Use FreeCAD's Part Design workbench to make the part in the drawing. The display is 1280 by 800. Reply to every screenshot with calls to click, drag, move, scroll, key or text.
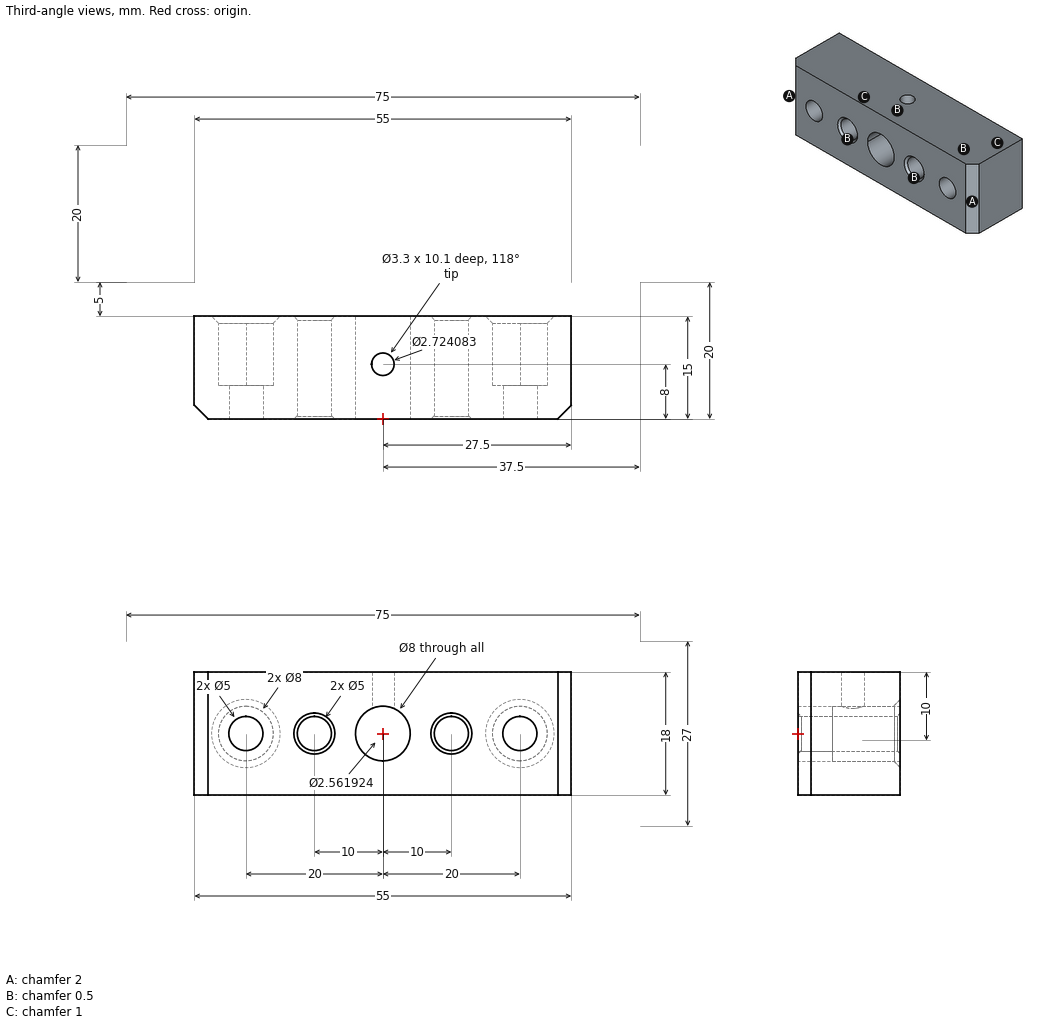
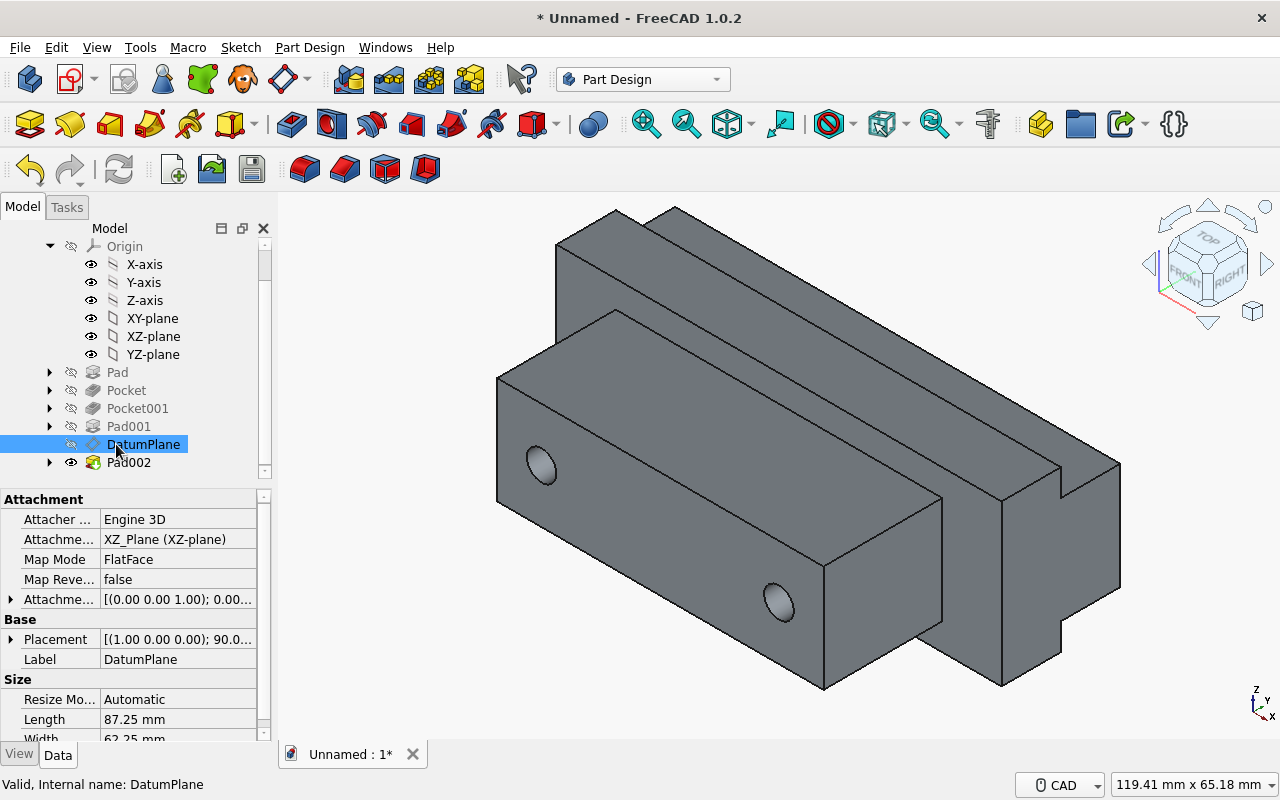
click(648, 124)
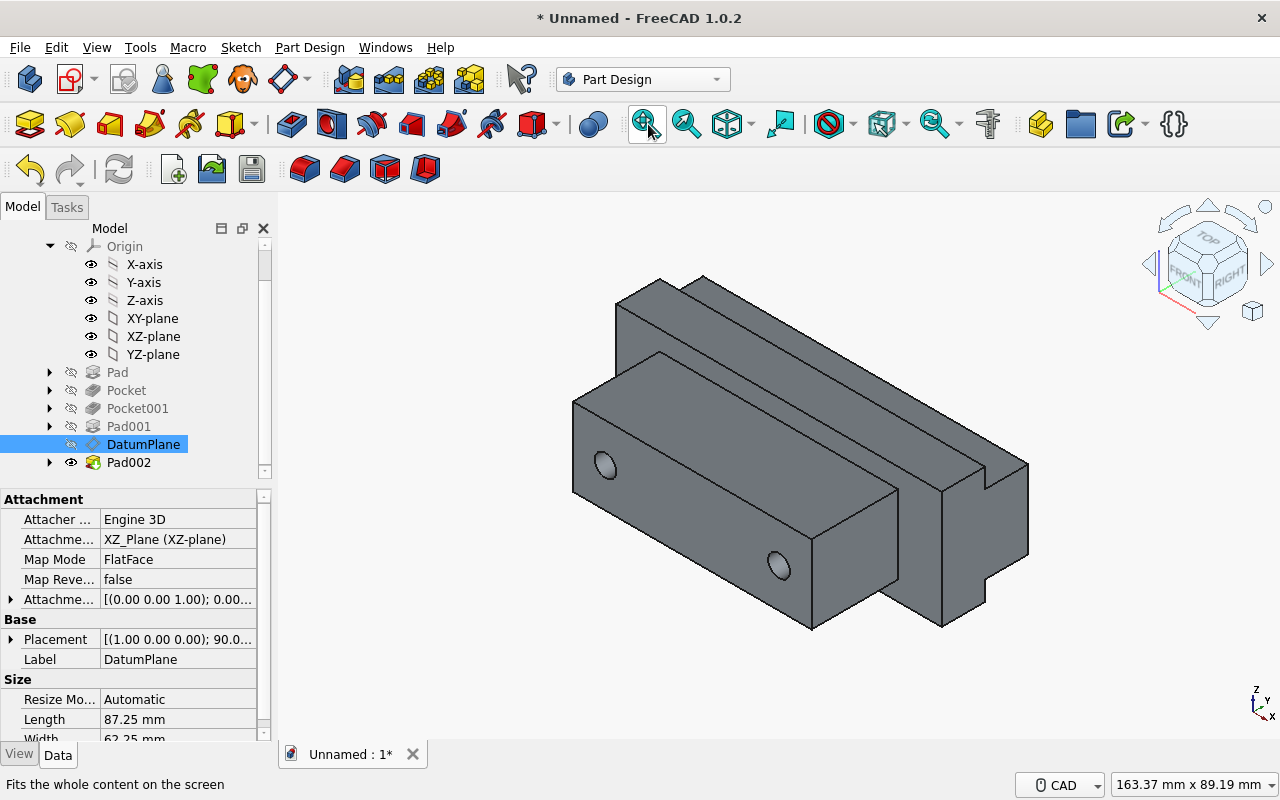
click(940, 465)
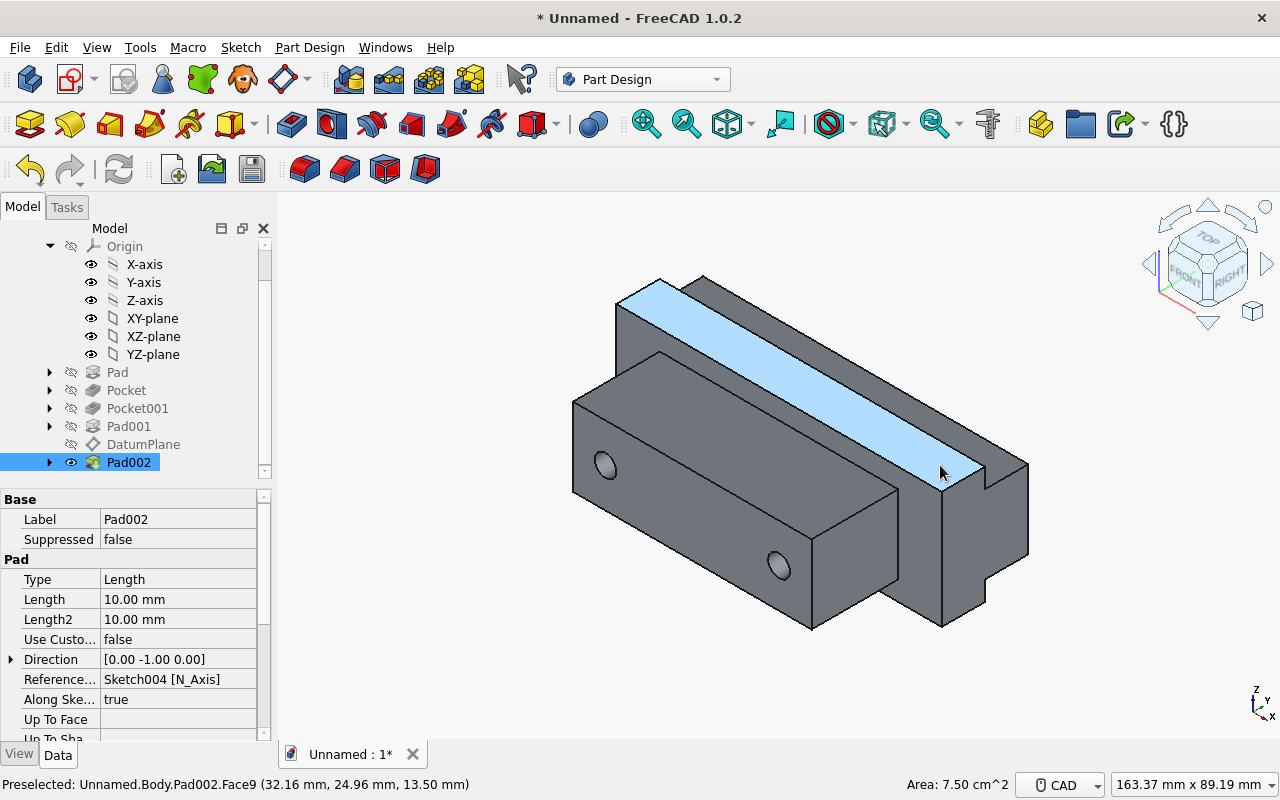
click(70, 80)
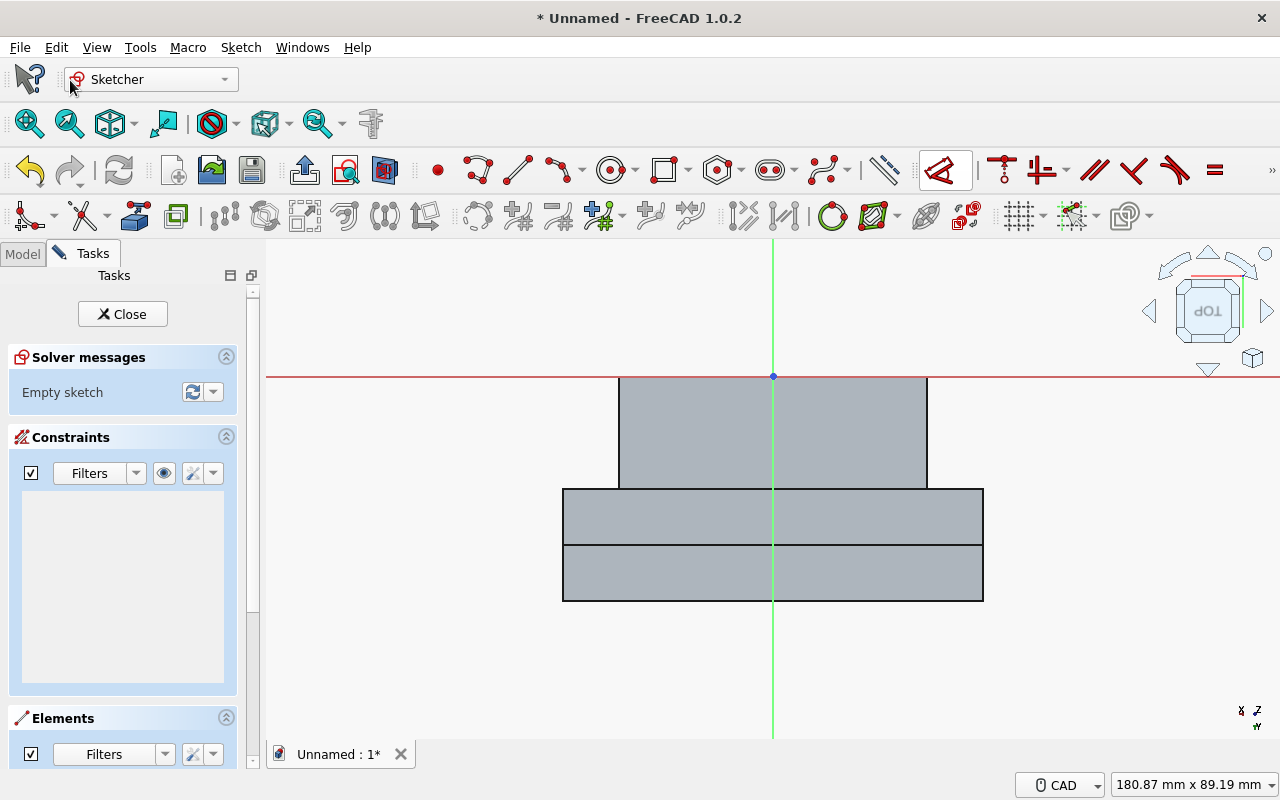
scroll(912, 489, up, 2)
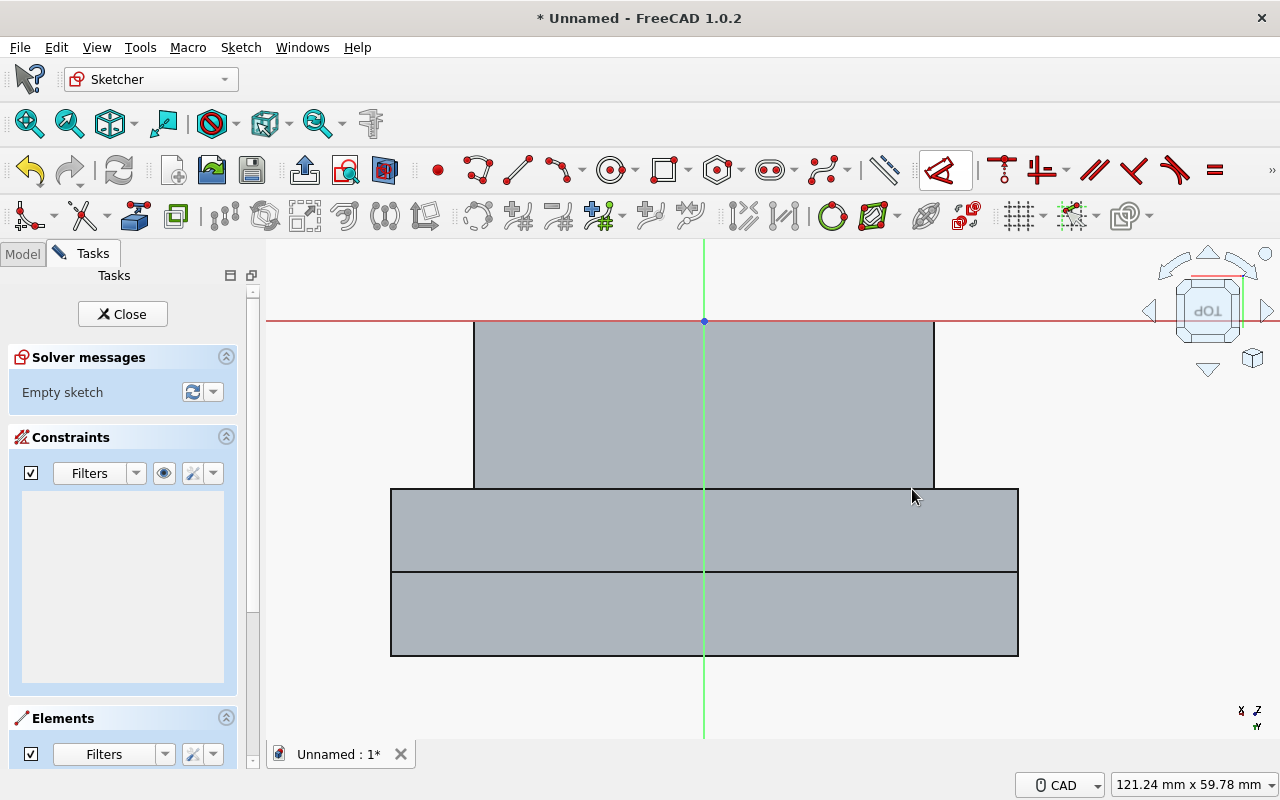
click(664, 170)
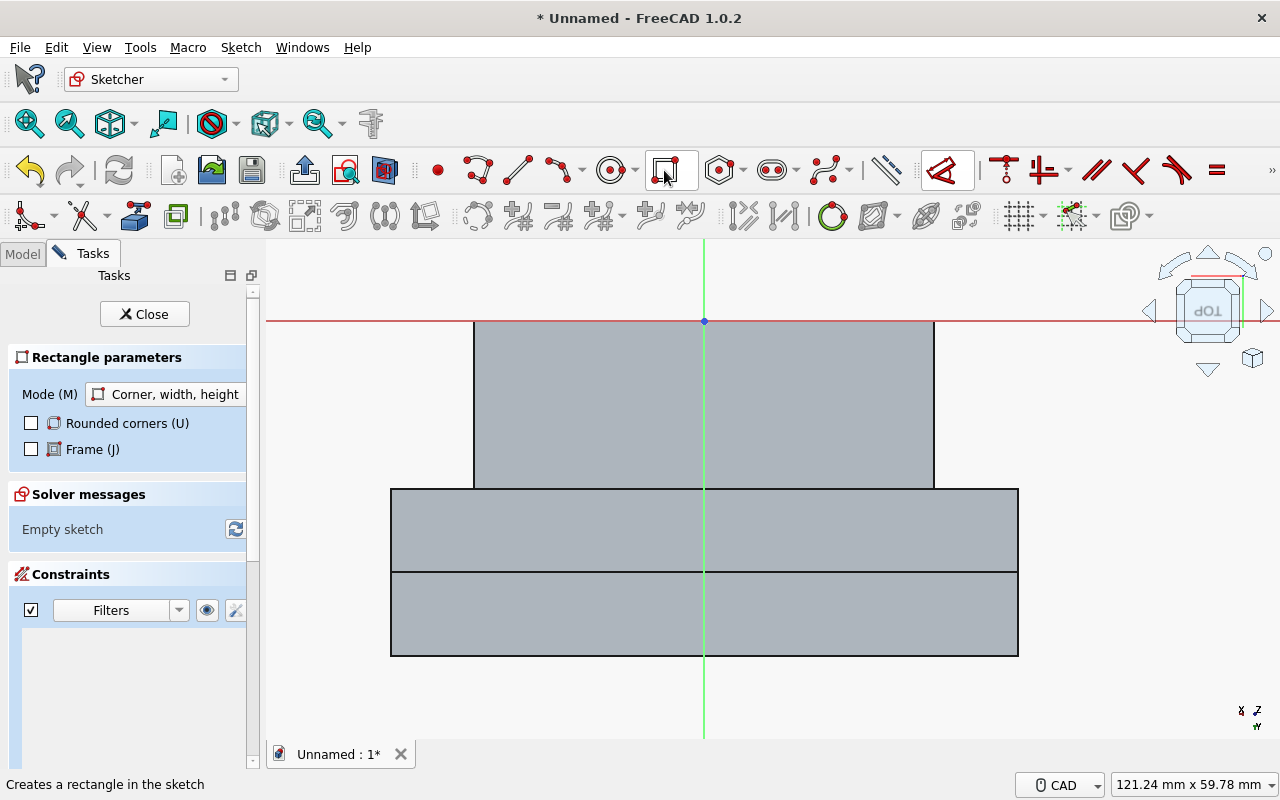
click(391, 489)
move(1018, 656)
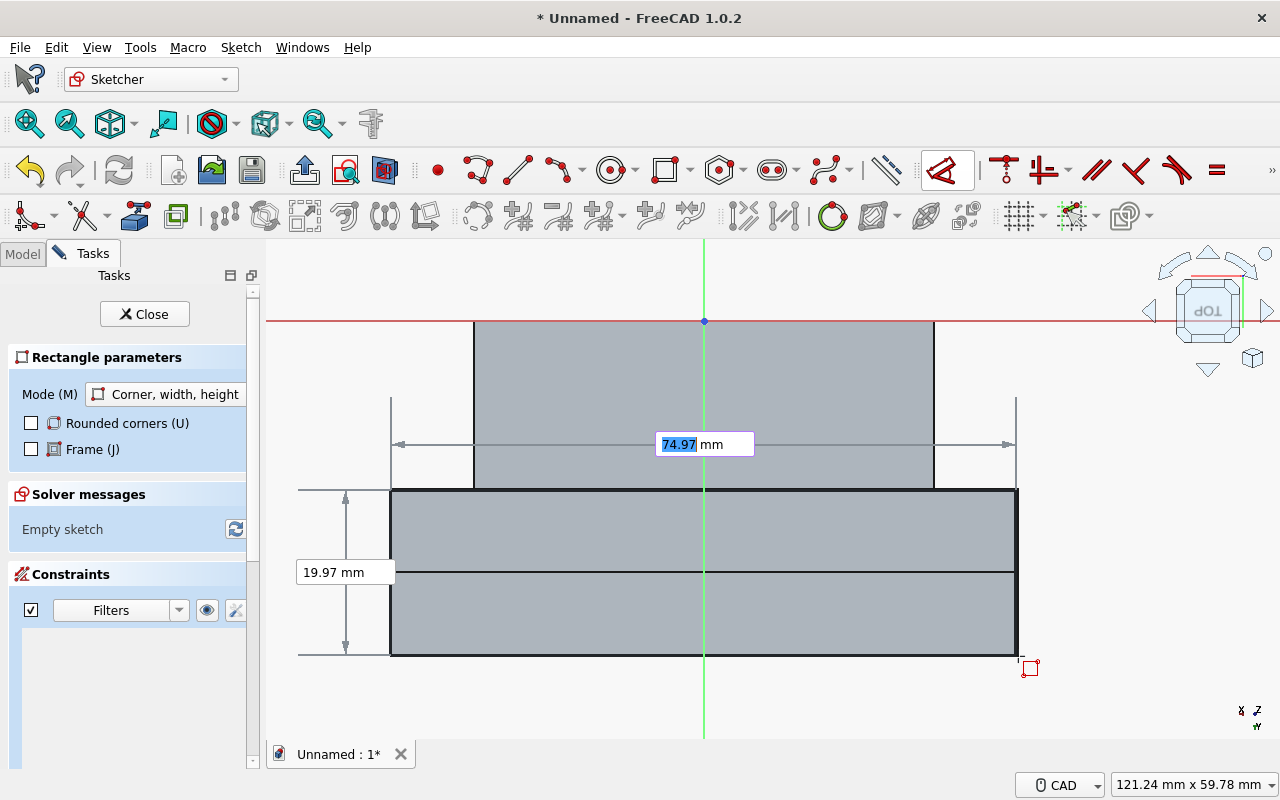
text(75)
key(Tab)
text(20)
key(Return)
key(Escape)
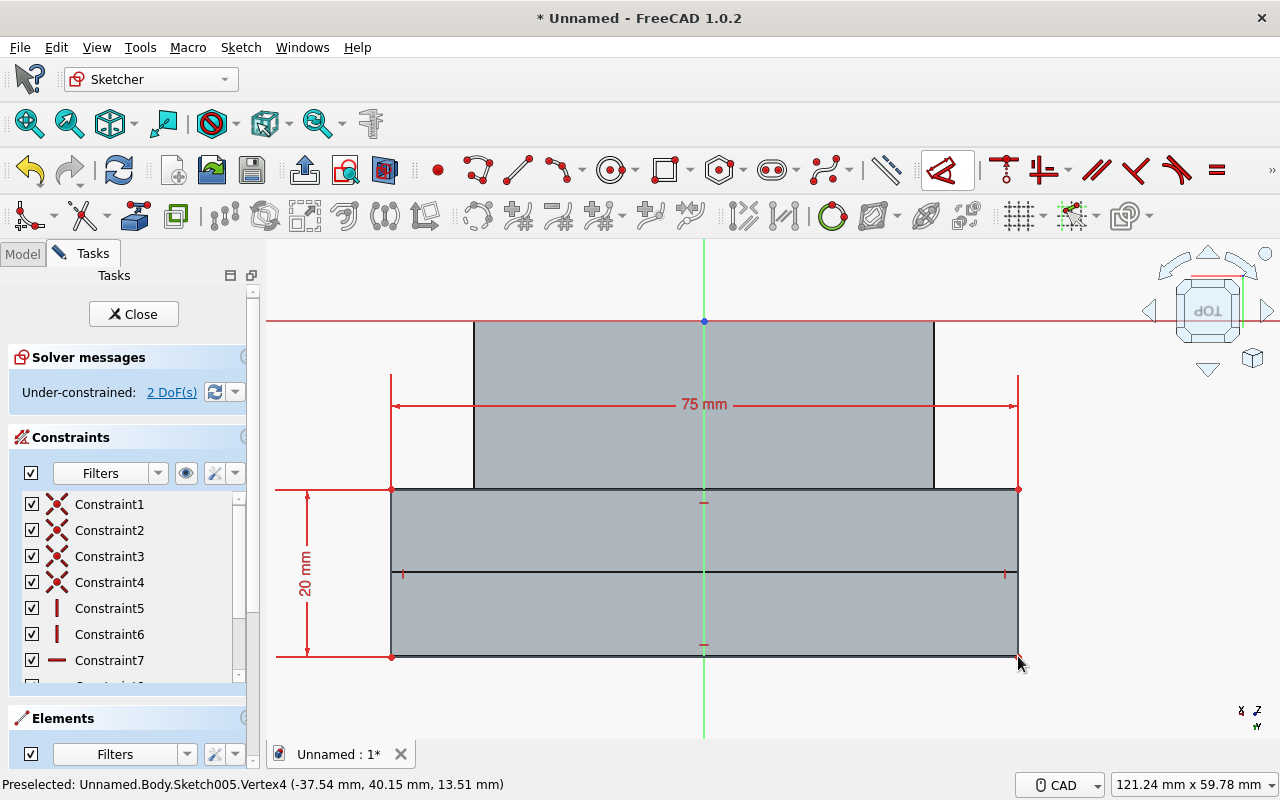
click(391, 490)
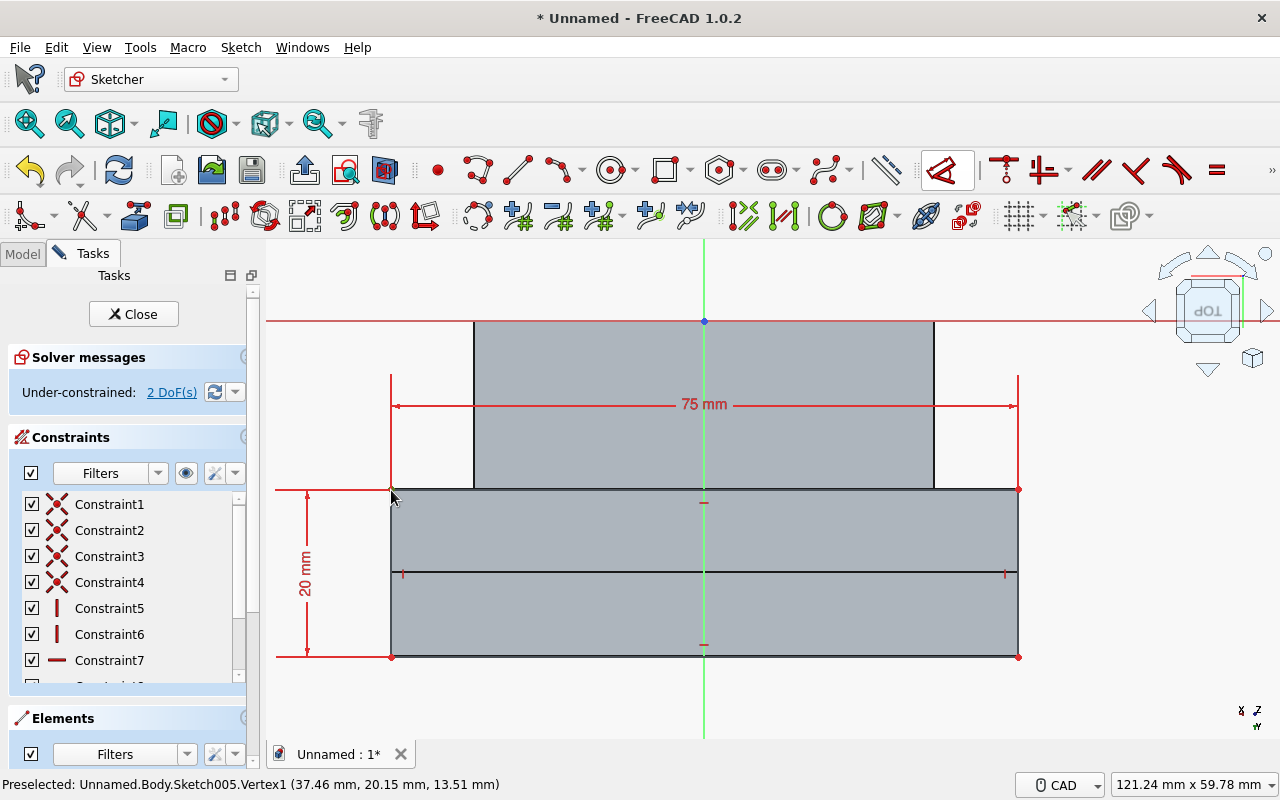
click(968, 170)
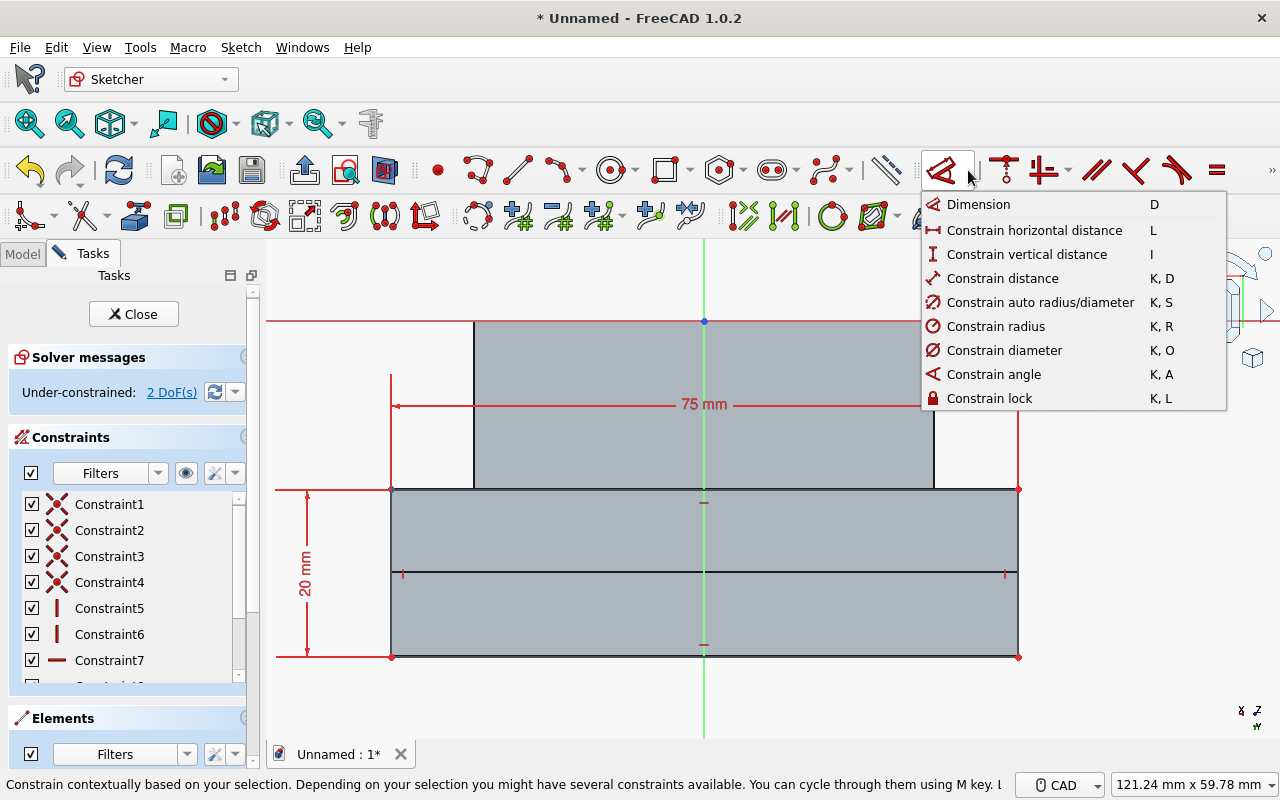
click(1074, 254)